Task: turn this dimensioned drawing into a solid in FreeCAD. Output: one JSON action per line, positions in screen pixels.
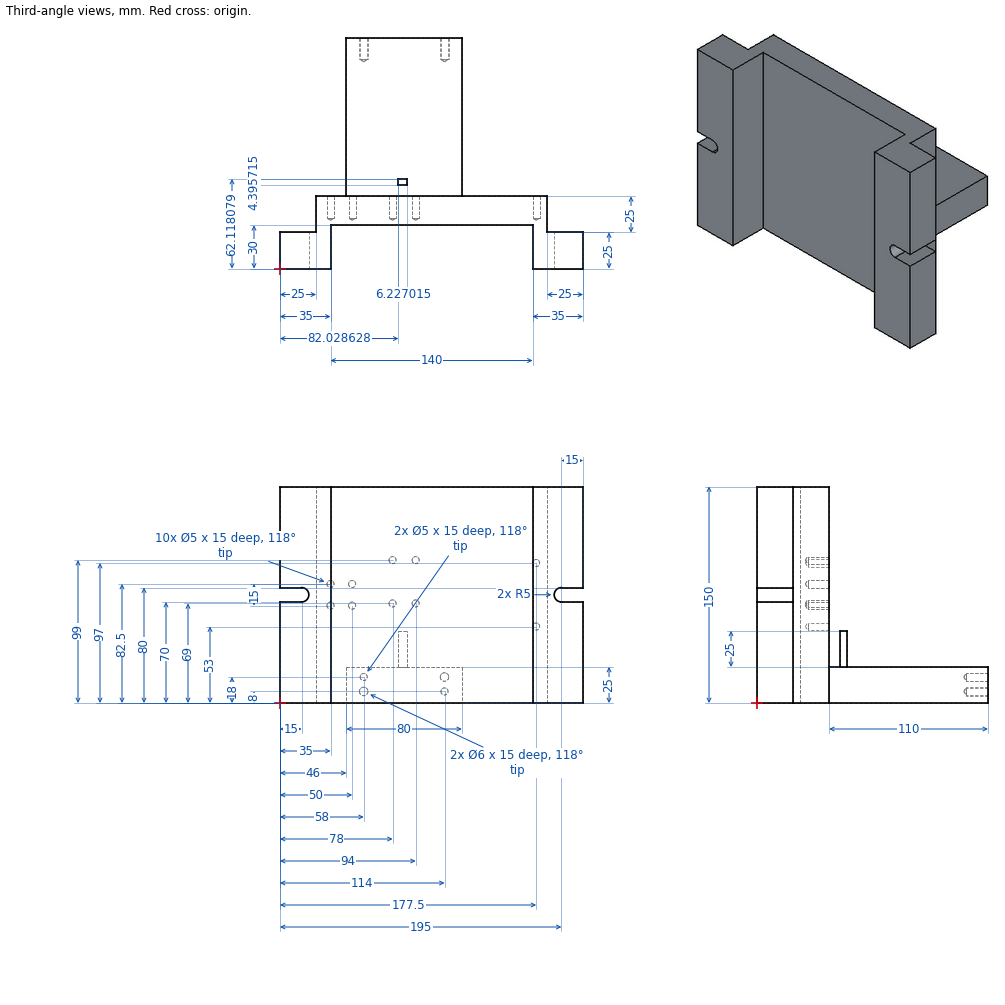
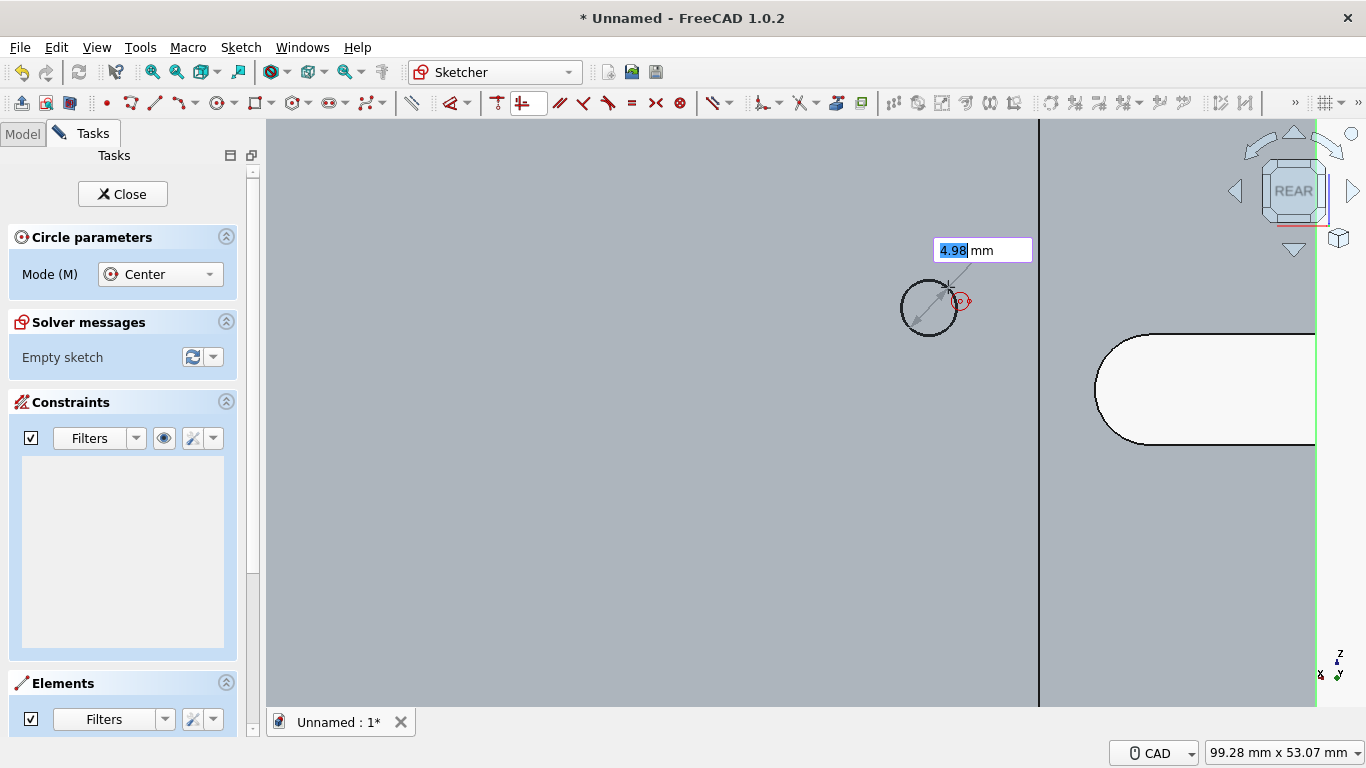
{"action": "type", "text": "5"}
{"action": "key", "text": "Return"}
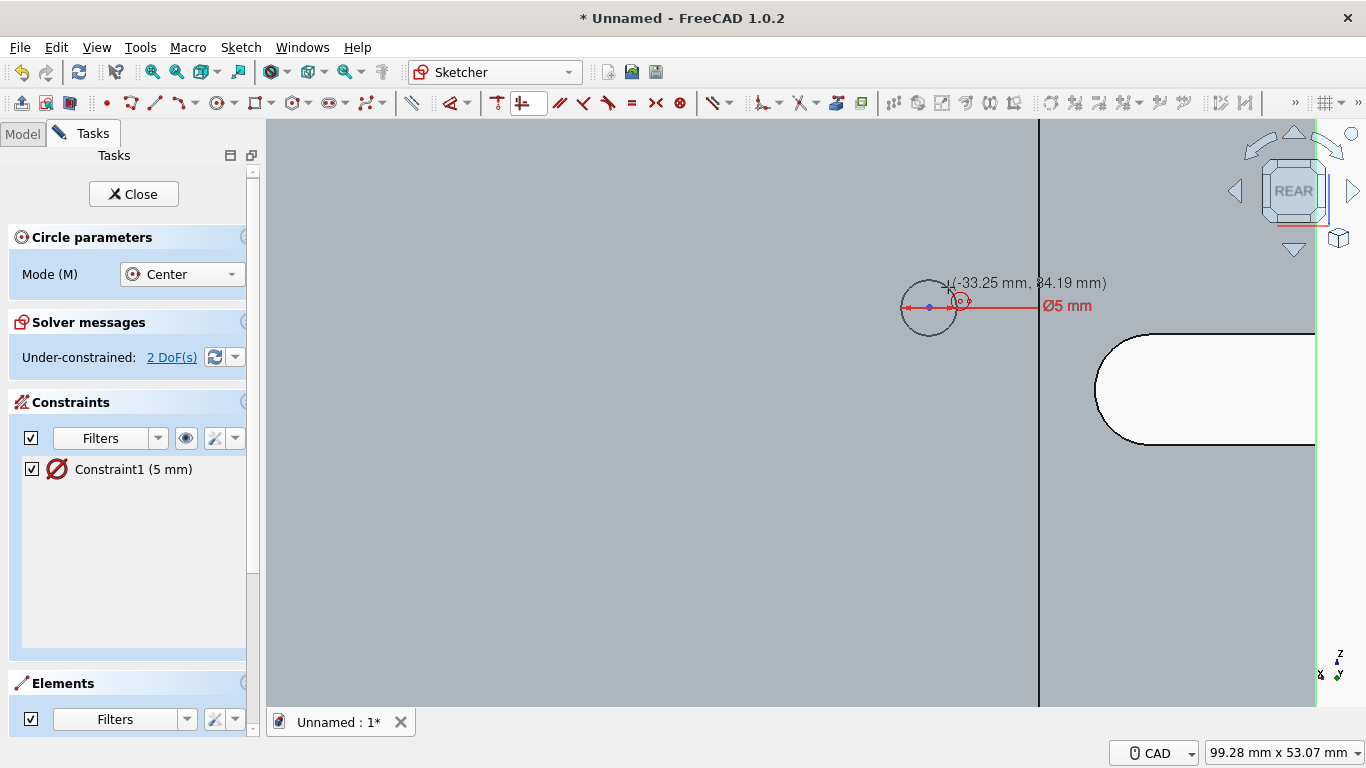
{"action": "left_click", "coordinate": [929, 473]}
{"action": "mouse_move", "coordinate": [948, 453]}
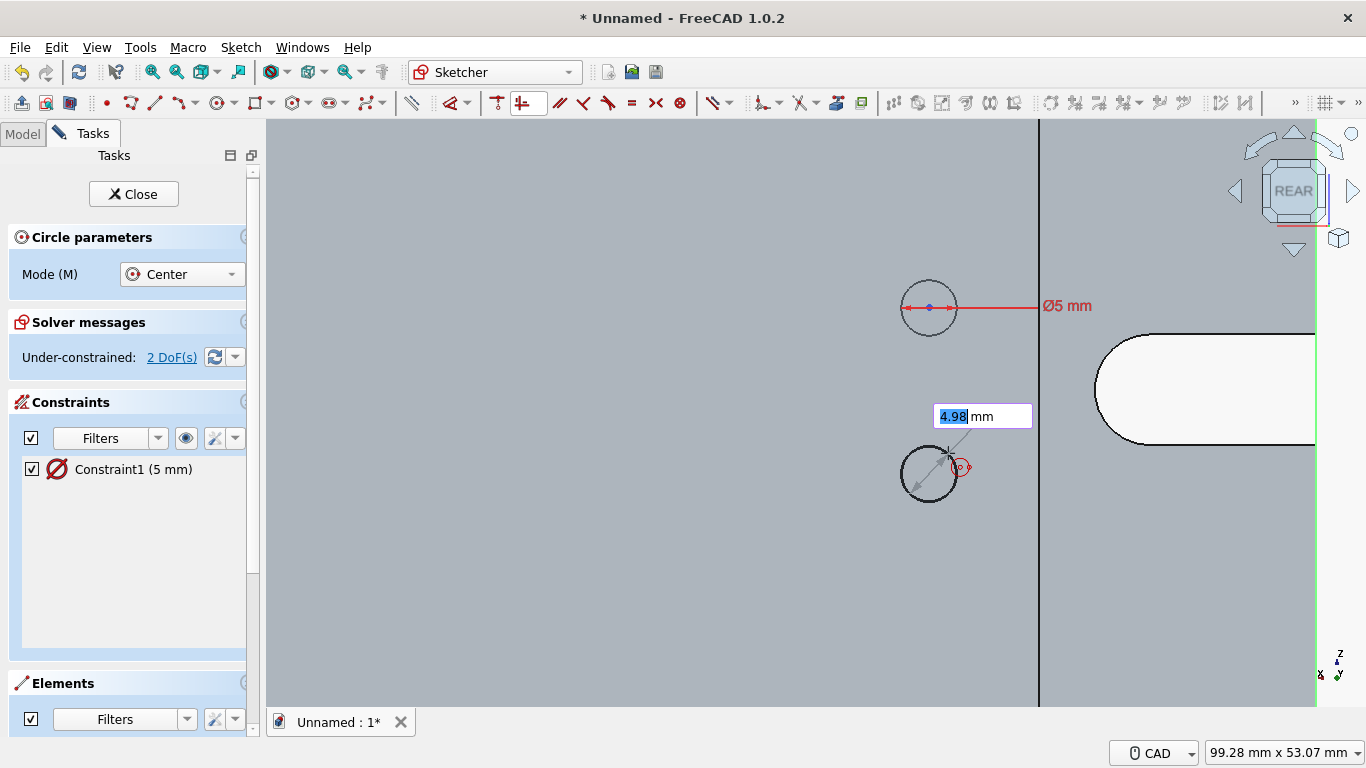
{"action": "type", "text": "5"}
{"action": "key", "text": "Return"}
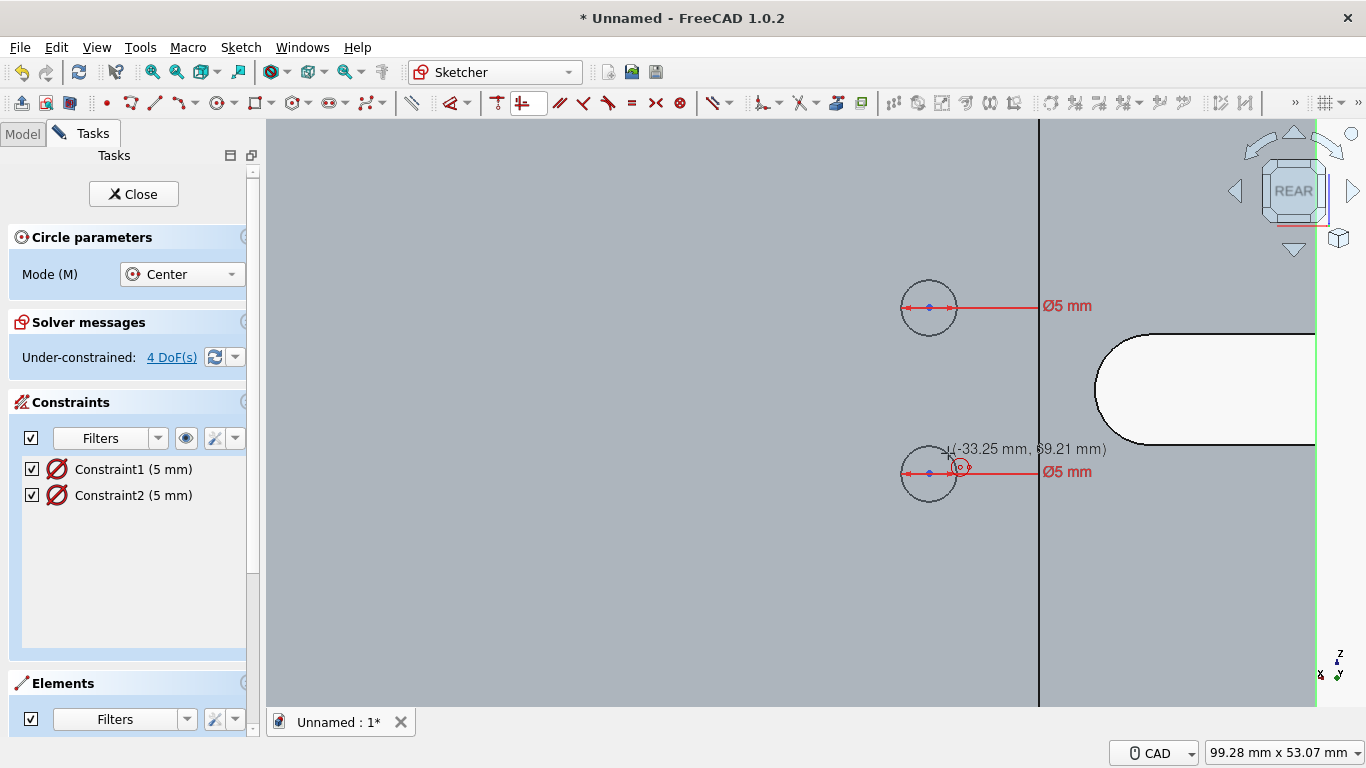
{"action": "left_click", "coordinate": [762, 473]}
{"action": "mouse_move", "coordinate": [782, 453]}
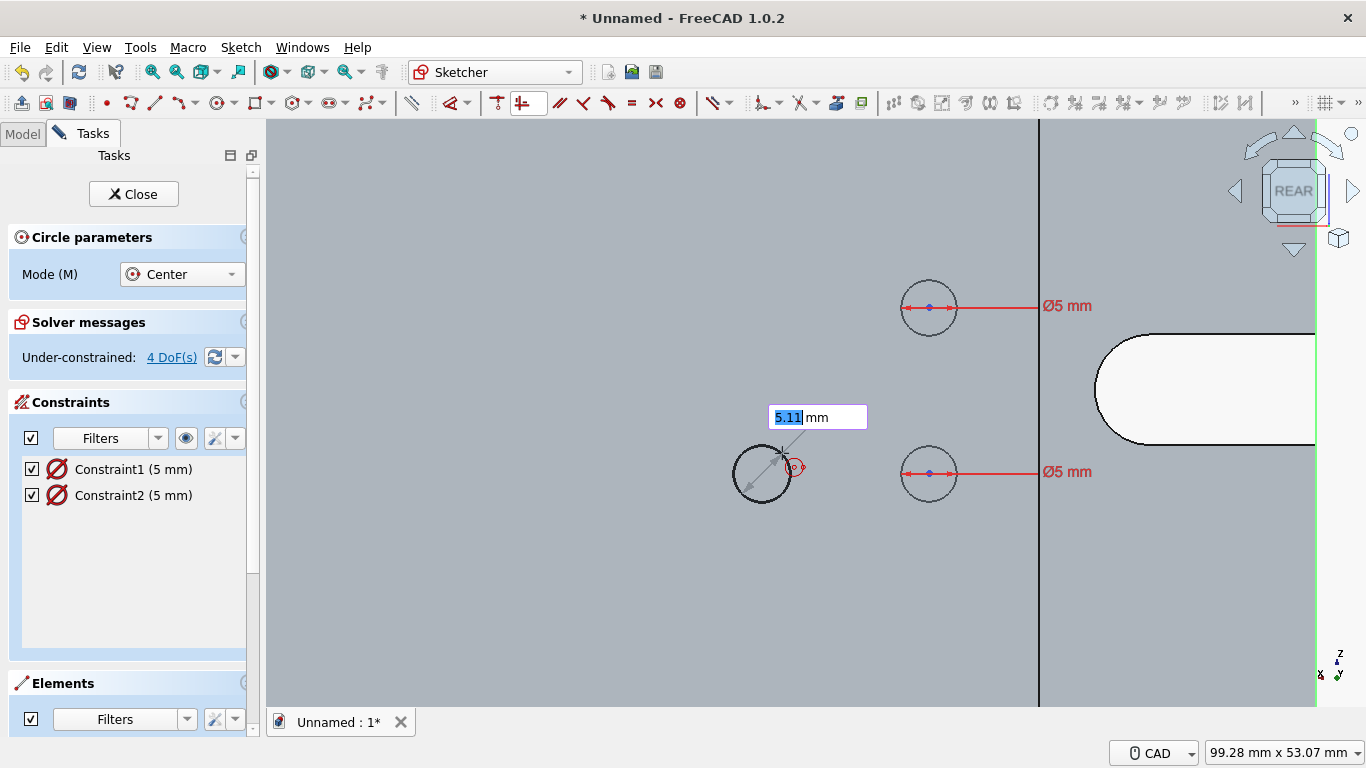
{"action": "type", "text": "5"}
{"action": "key", "text": "Return"}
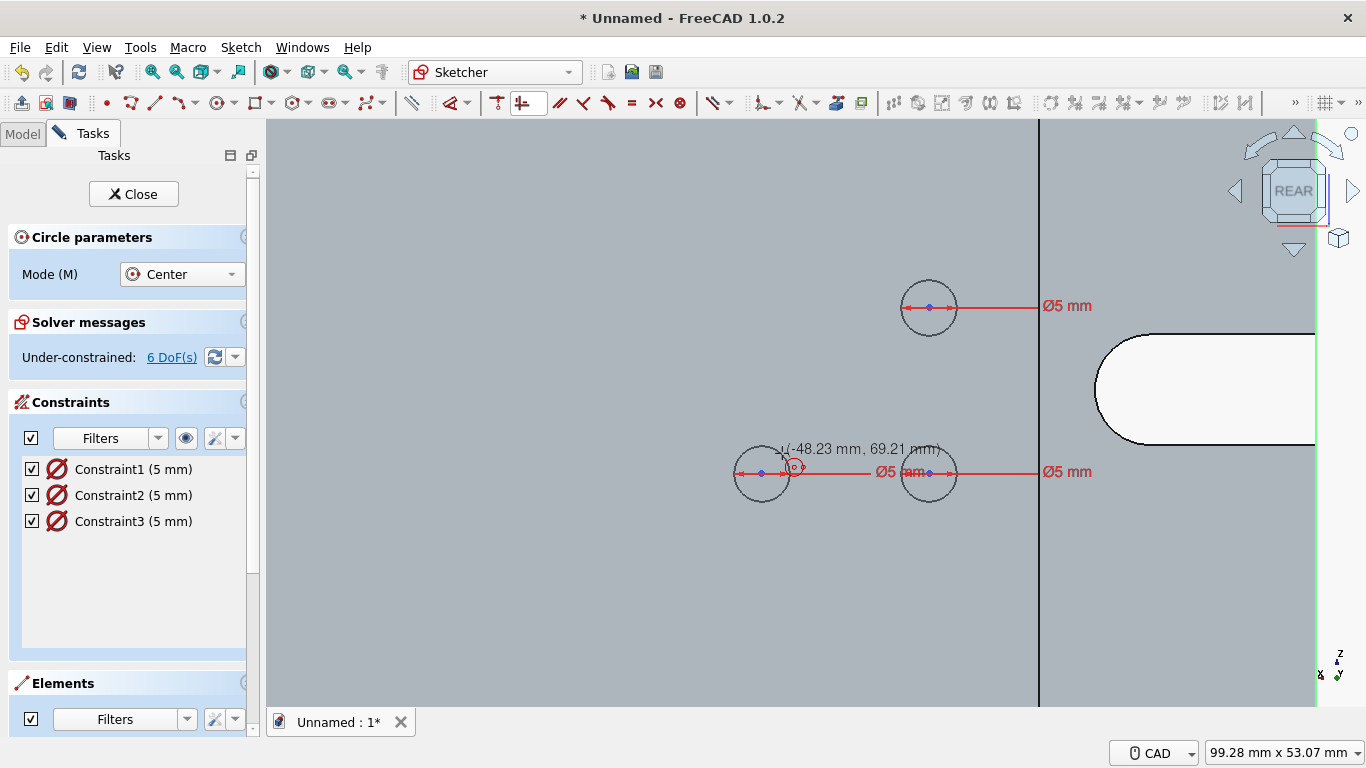
{"action": "left_click", "coordinate": [762, 307]}
{"action": "mouse_move", "coordinate": [782, 287]}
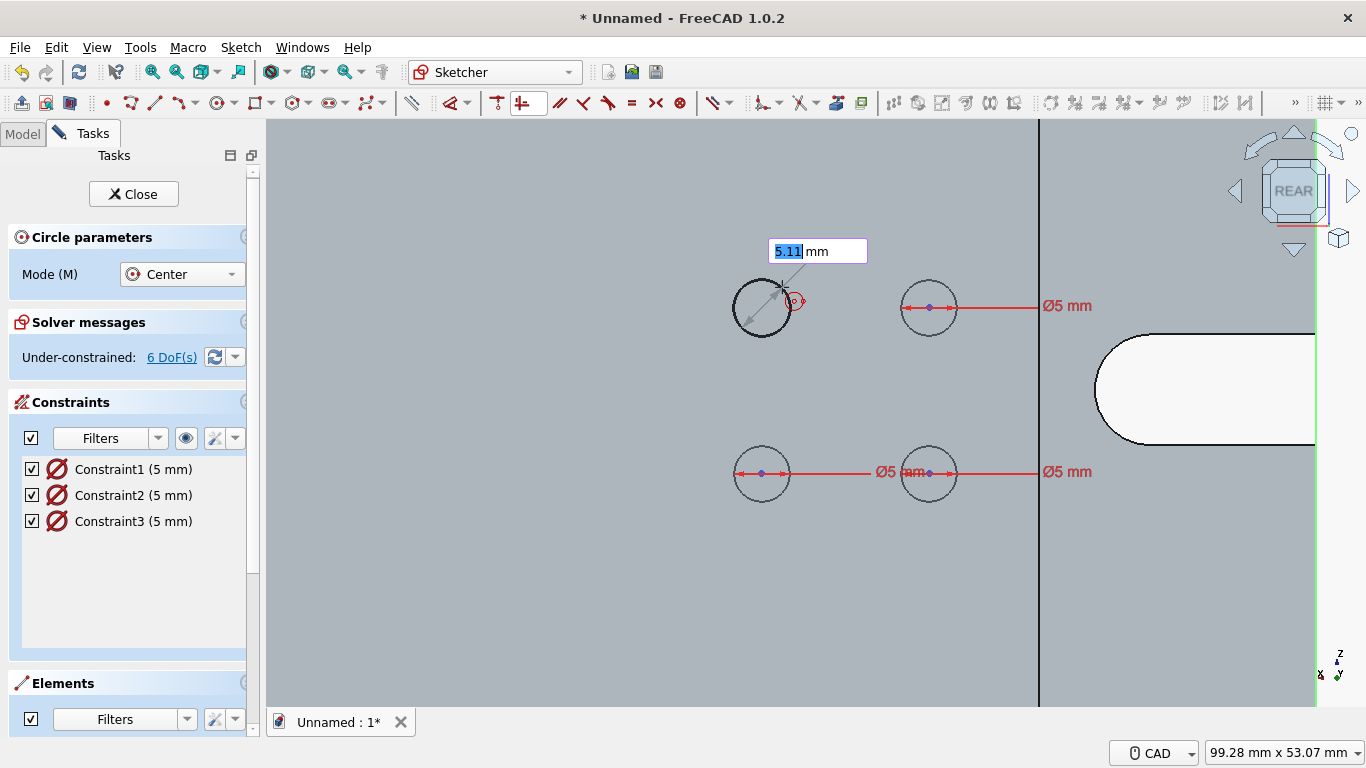
{"action": "type", "text": "5"}
{"action": "key", "text": "Return"}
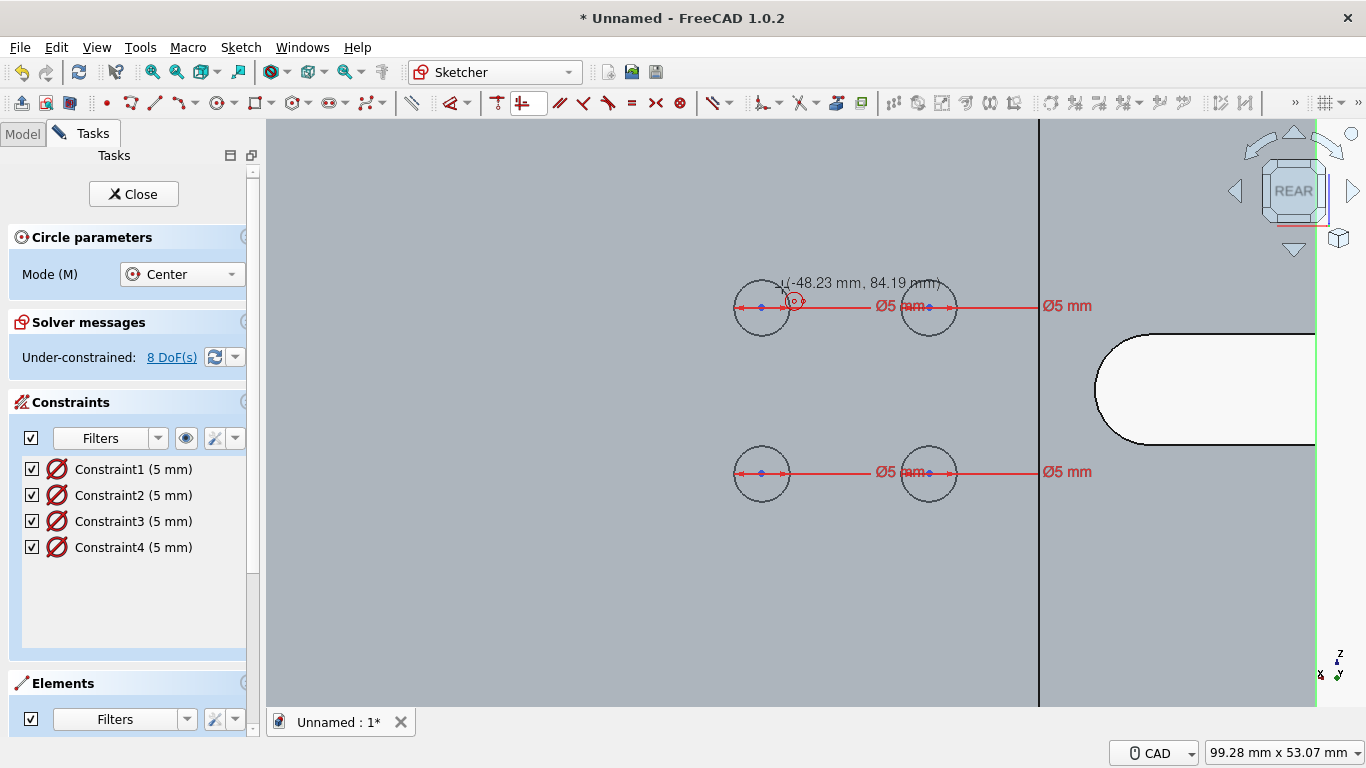
{"action": "left_click", "coordinate": [452, 456]}
{"action": "mouse_move", "coordinate": [472, 437]}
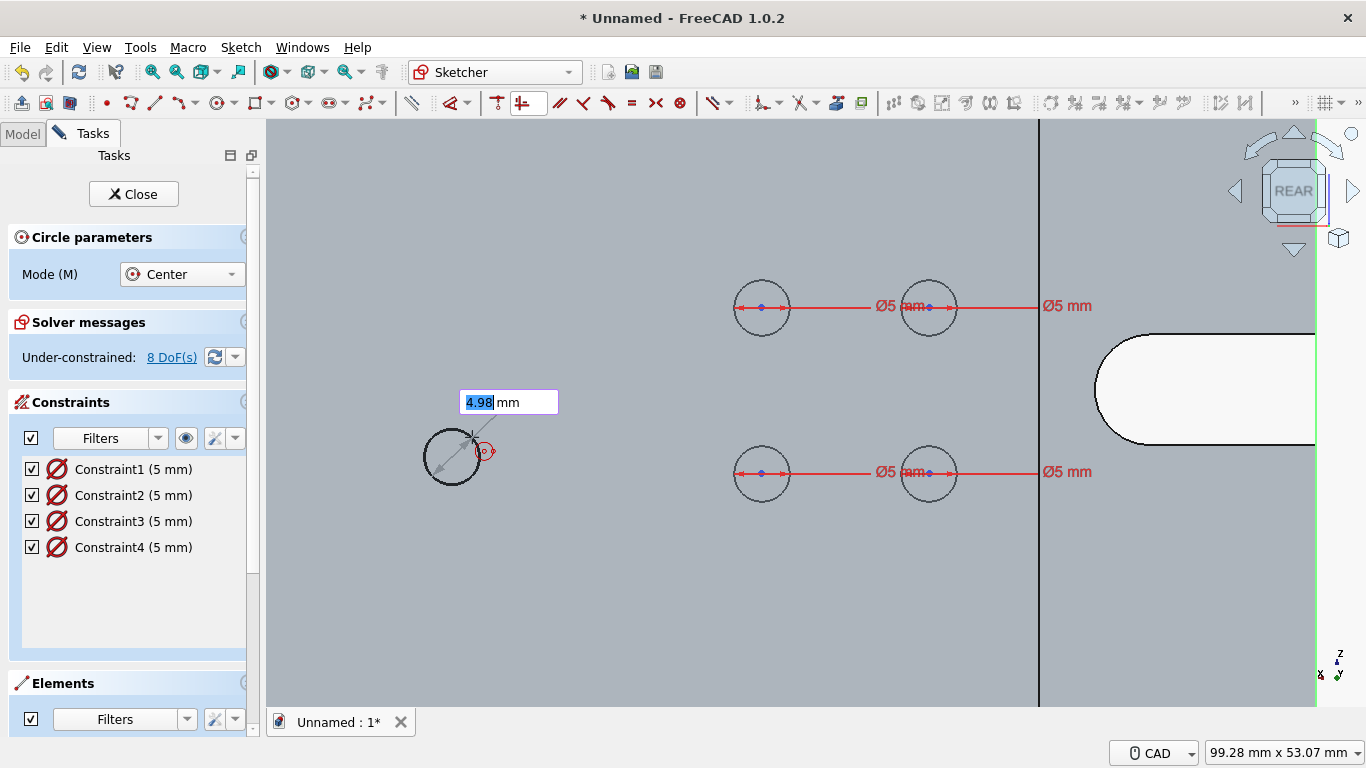
{"action": "type", "text": "5"}
{"action": "key", "text": "Return"}